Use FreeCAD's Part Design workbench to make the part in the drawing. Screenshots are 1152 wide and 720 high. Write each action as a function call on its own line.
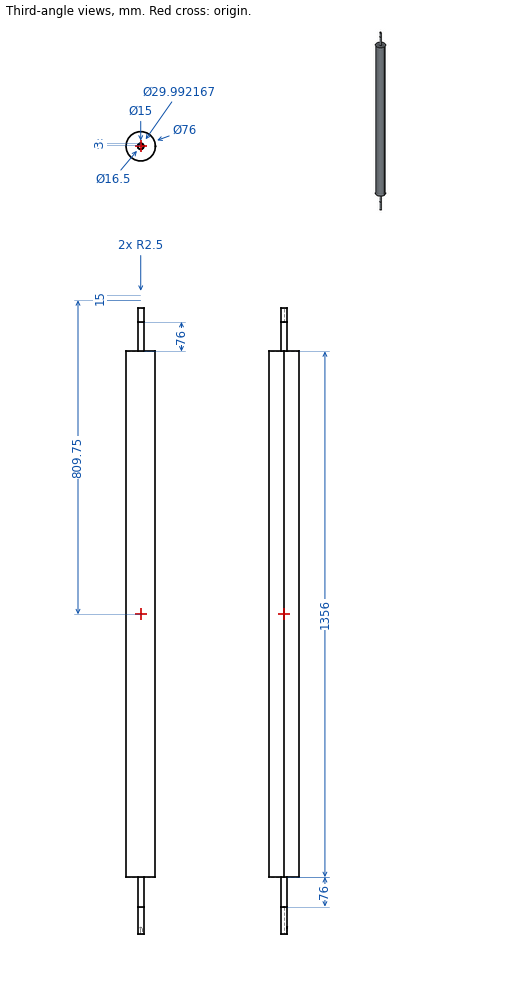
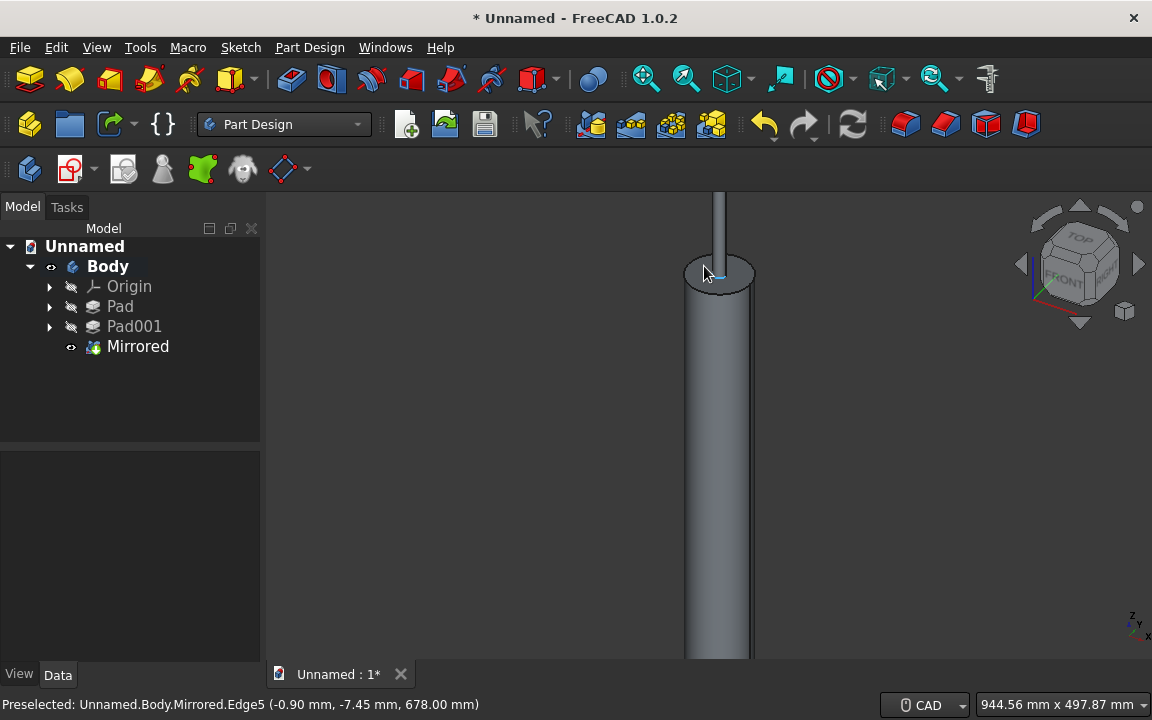
click(702, 267)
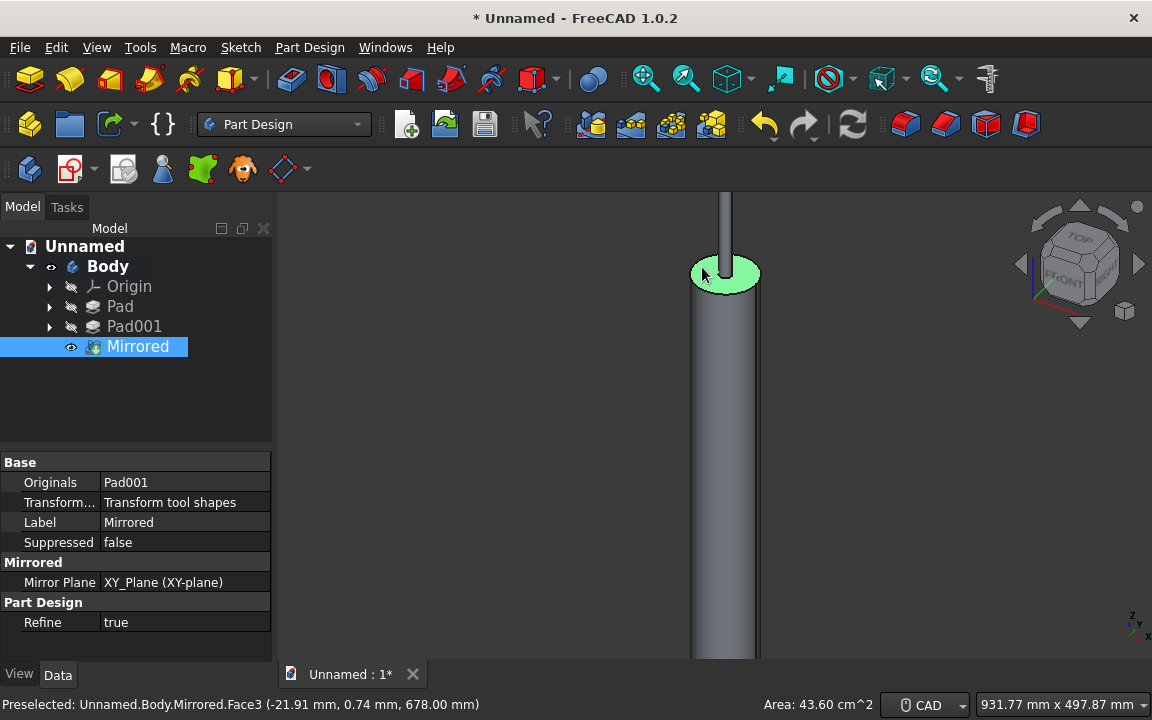
click(70, 170)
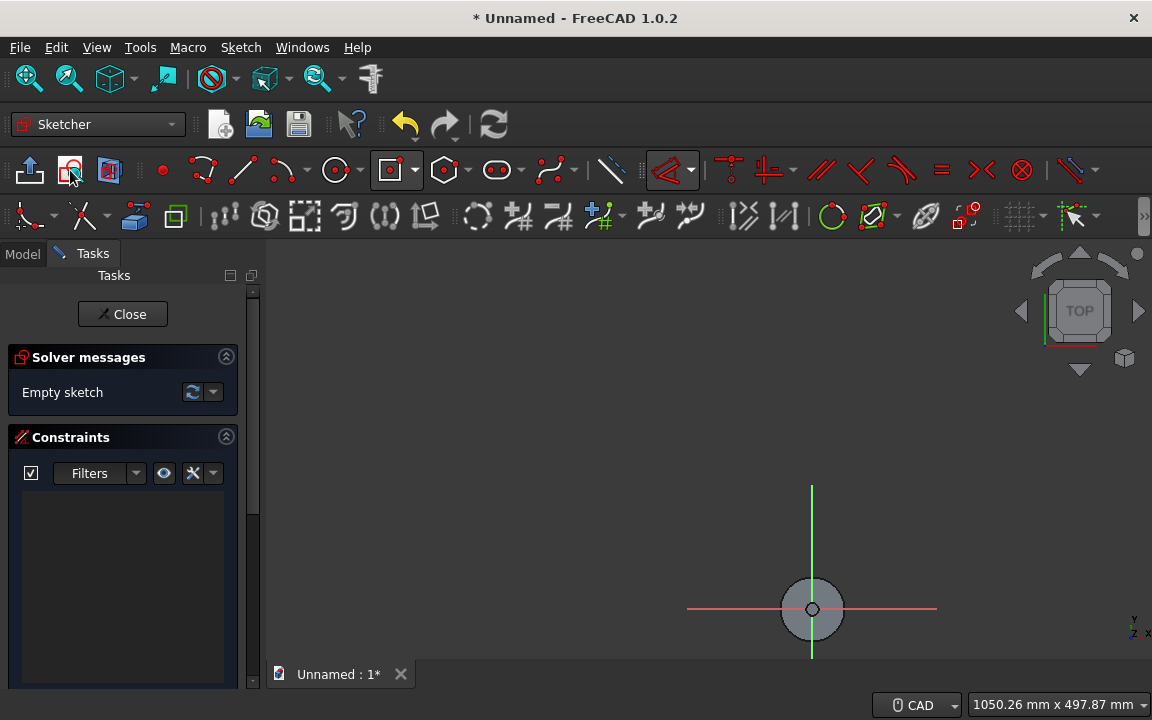
click(110, 170)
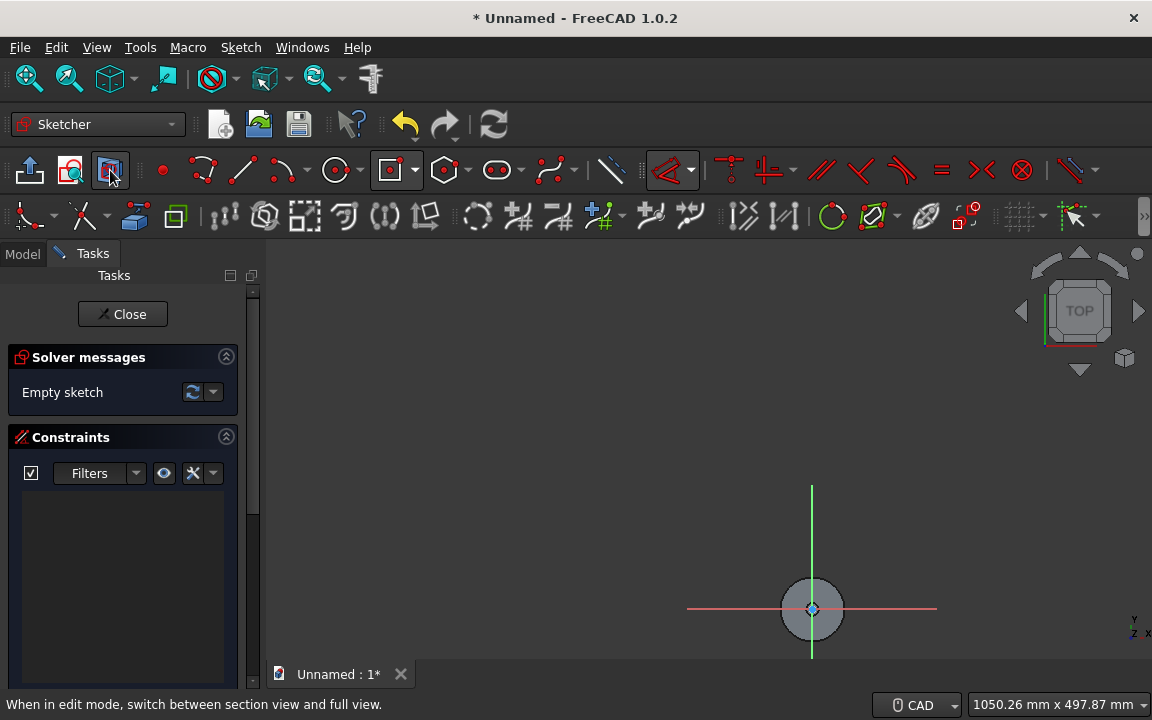
scroll(822, 618, up, 15)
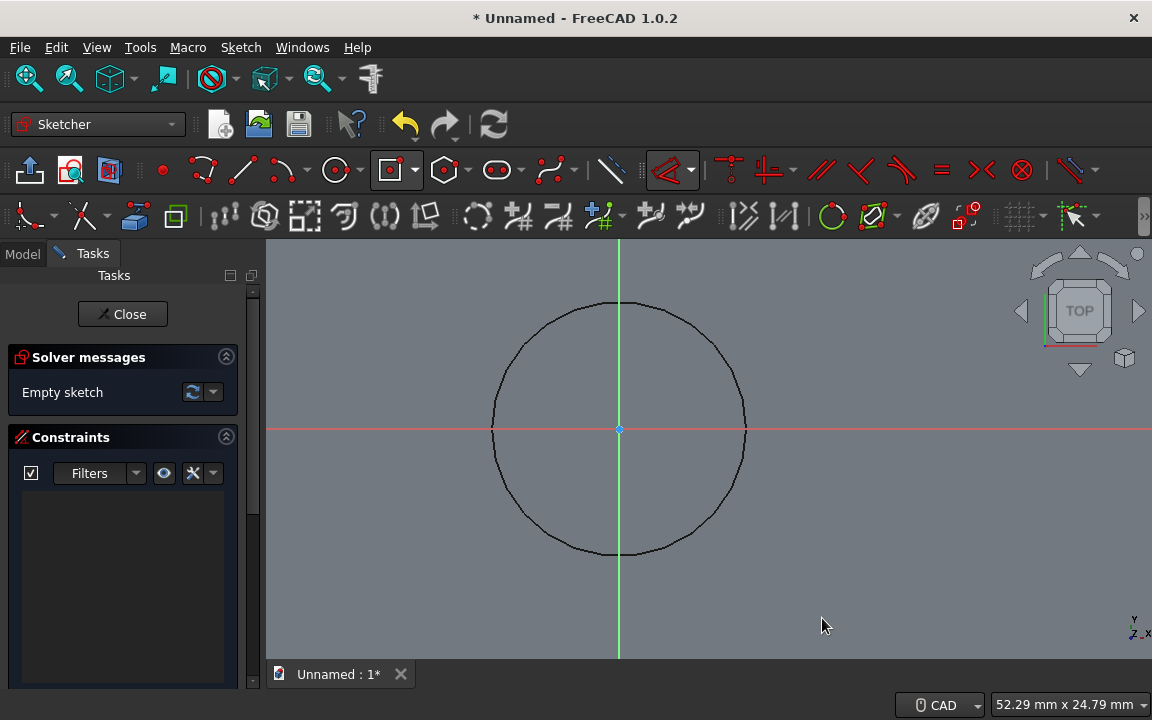
scroll(737, 539, down, 1)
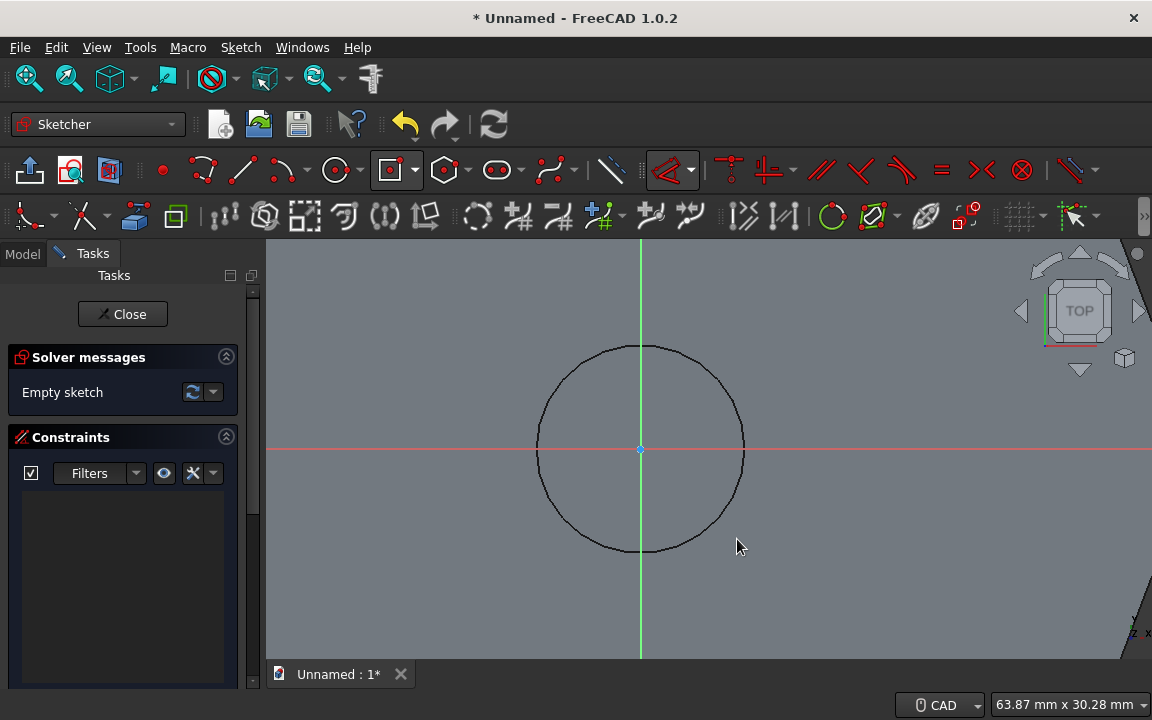
click(336, 170)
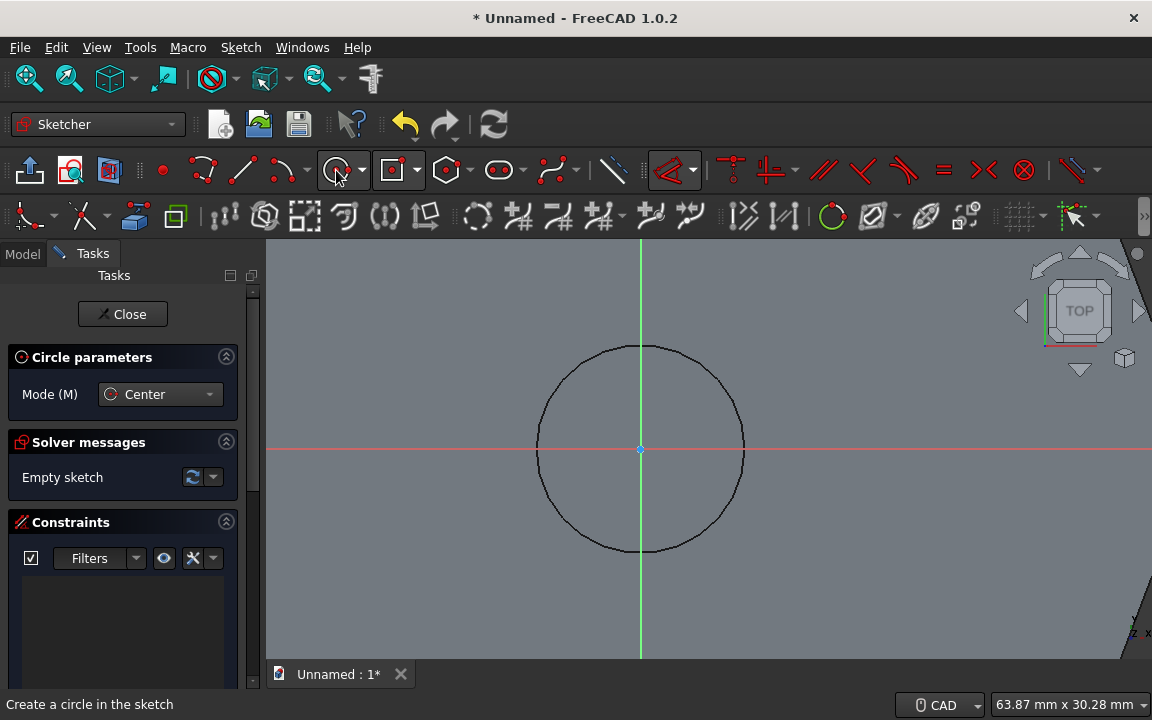
click(641, 449)
click(721, 368)
key(Escape)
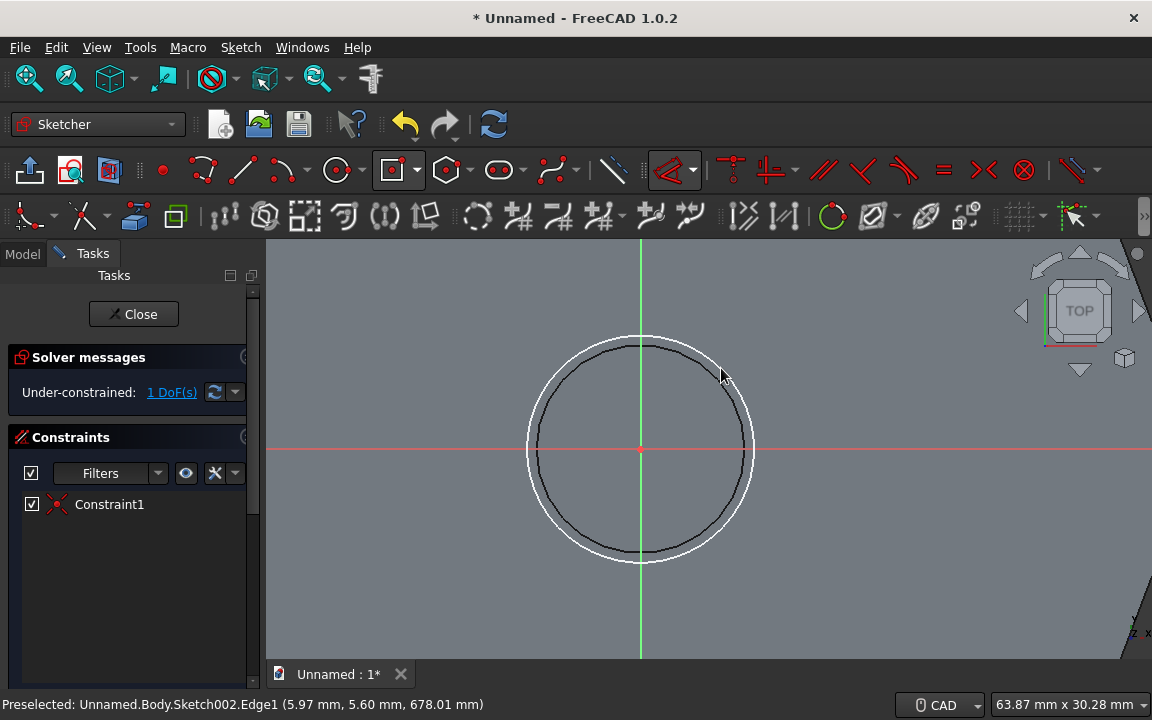
click(721, 369)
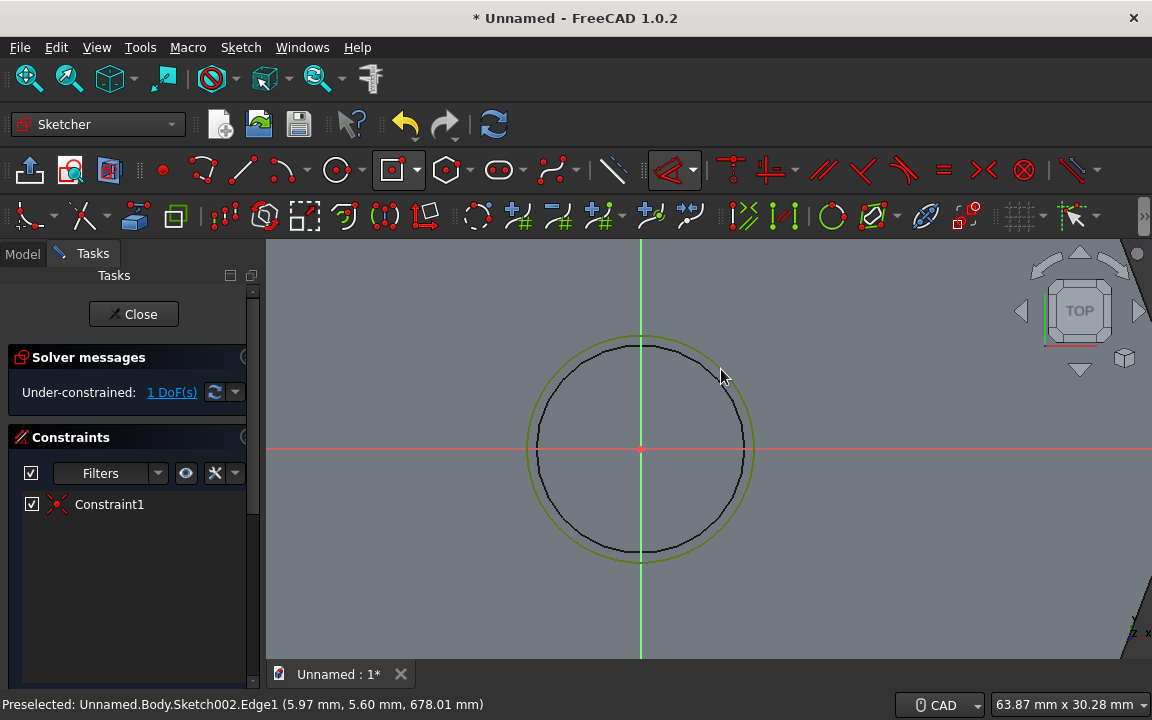
click(696, 170)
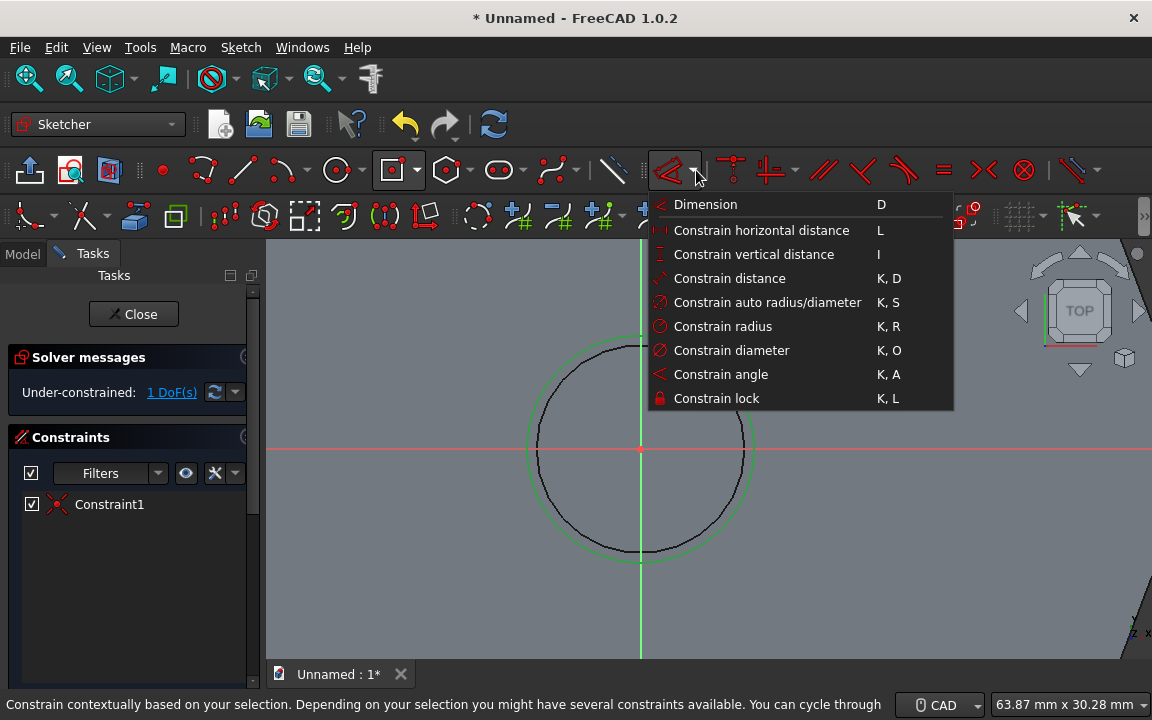
click(801, 350)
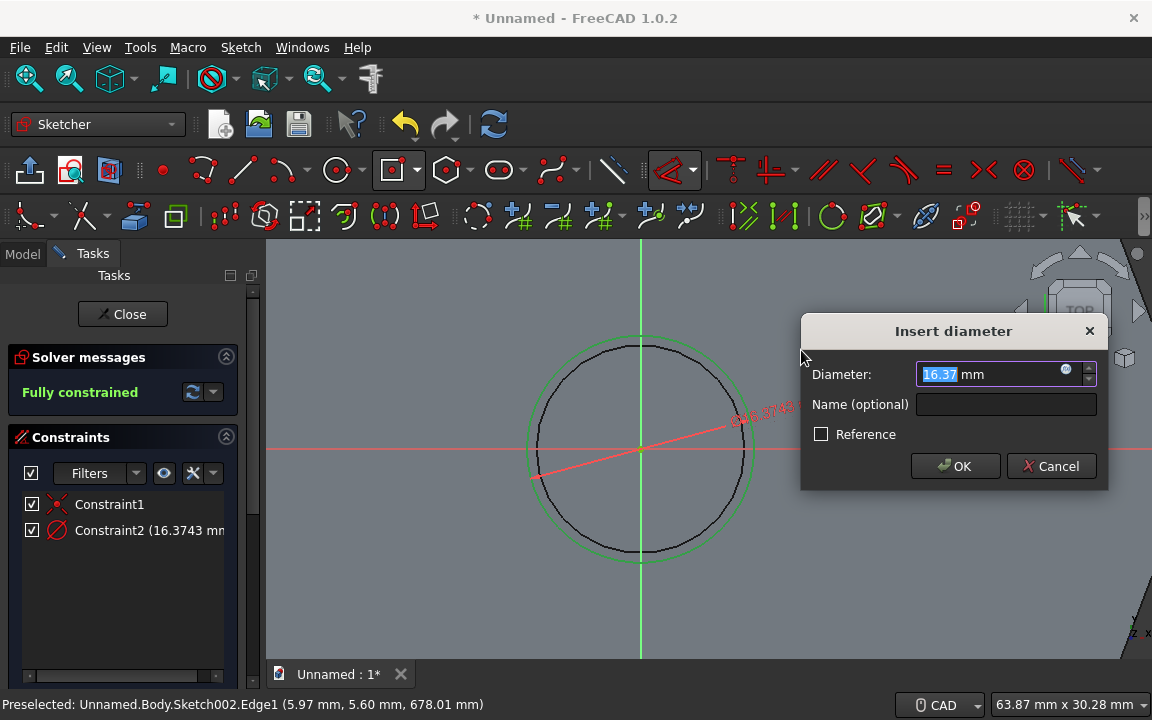
text(16.5)
key(Return)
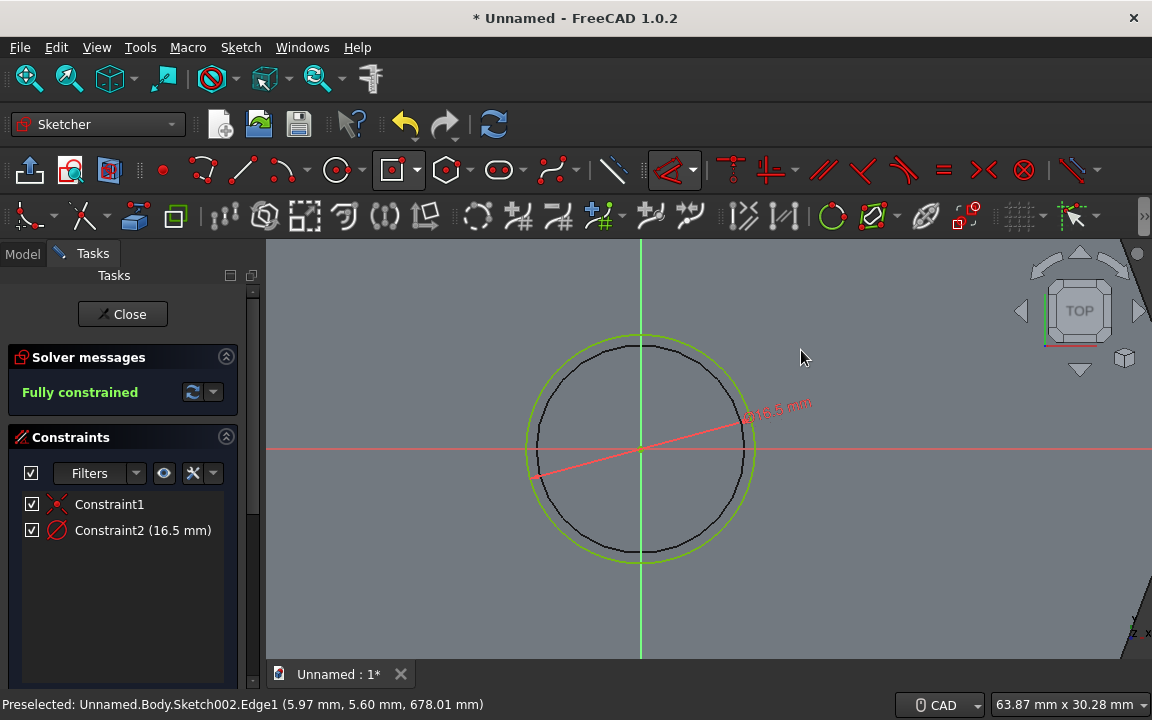
click(123, 314)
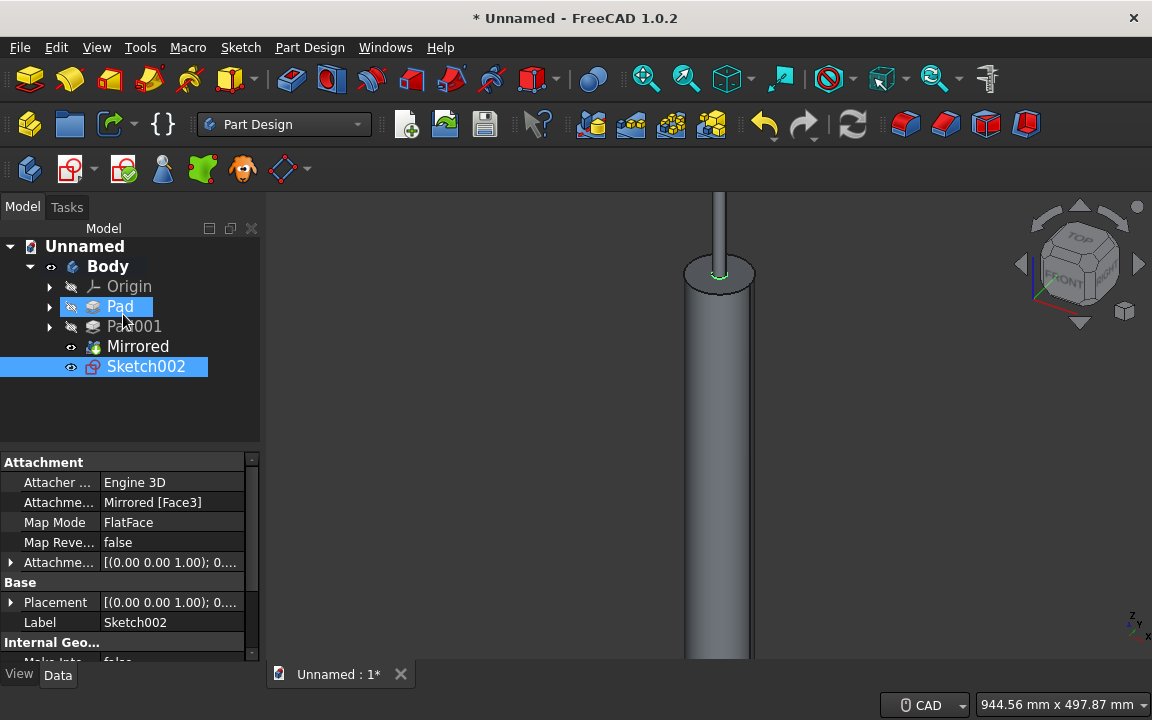
click(30, 80)